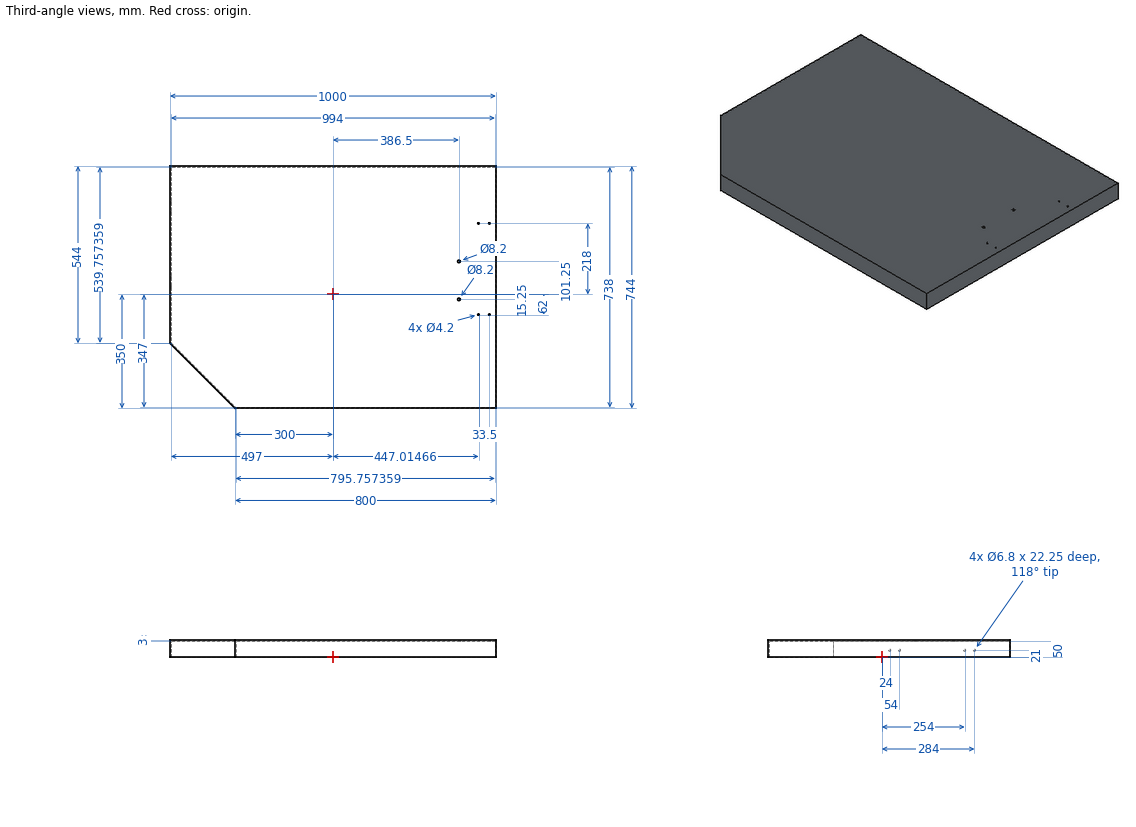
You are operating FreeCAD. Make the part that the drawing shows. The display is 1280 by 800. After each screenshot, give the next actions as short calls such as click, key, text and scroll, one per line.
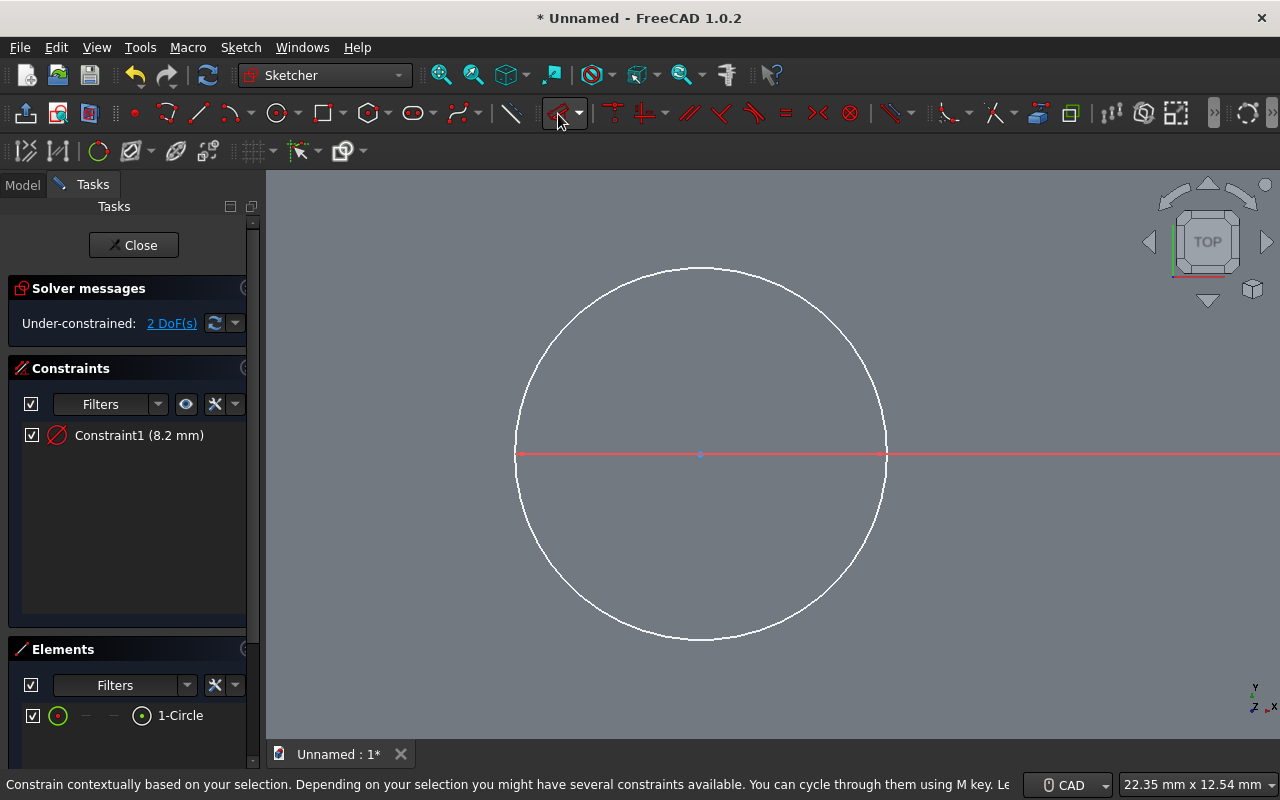
click(701, 454)
click(497, 420)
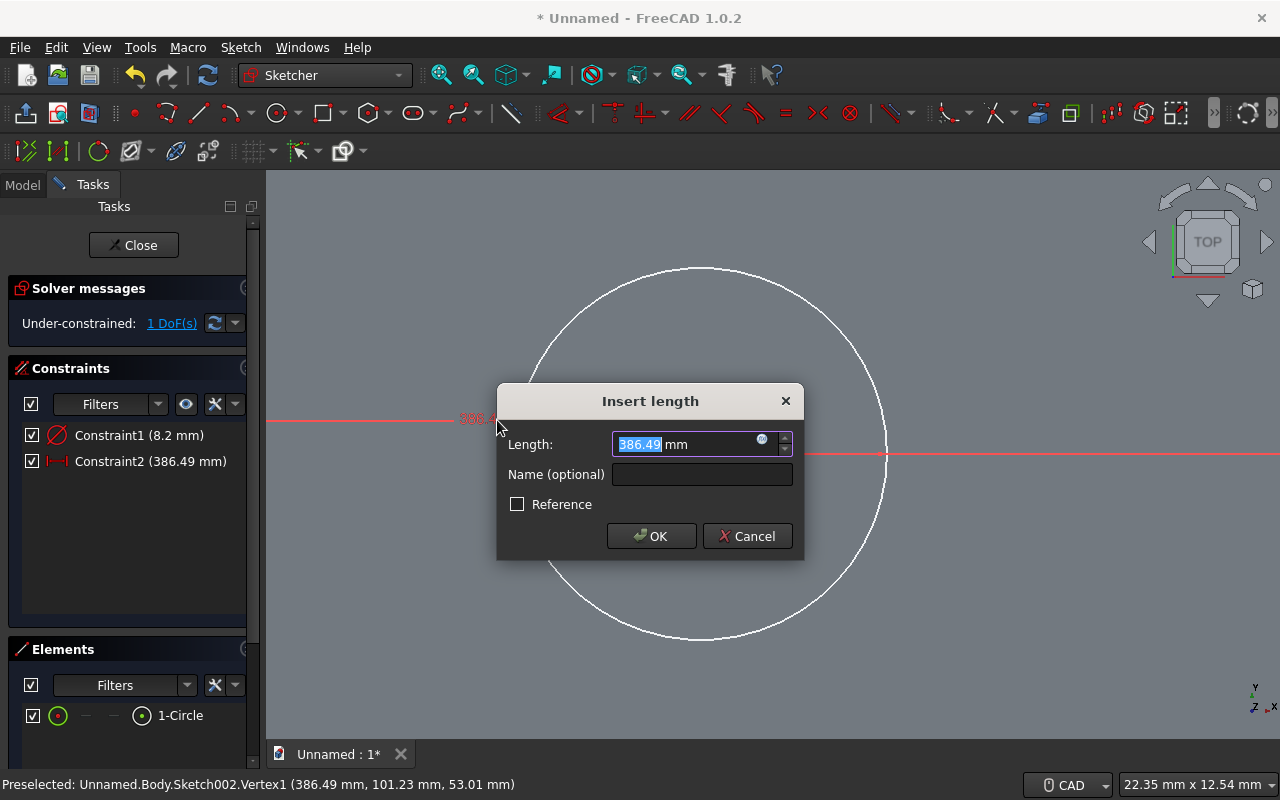
text(386.5)
key(Return)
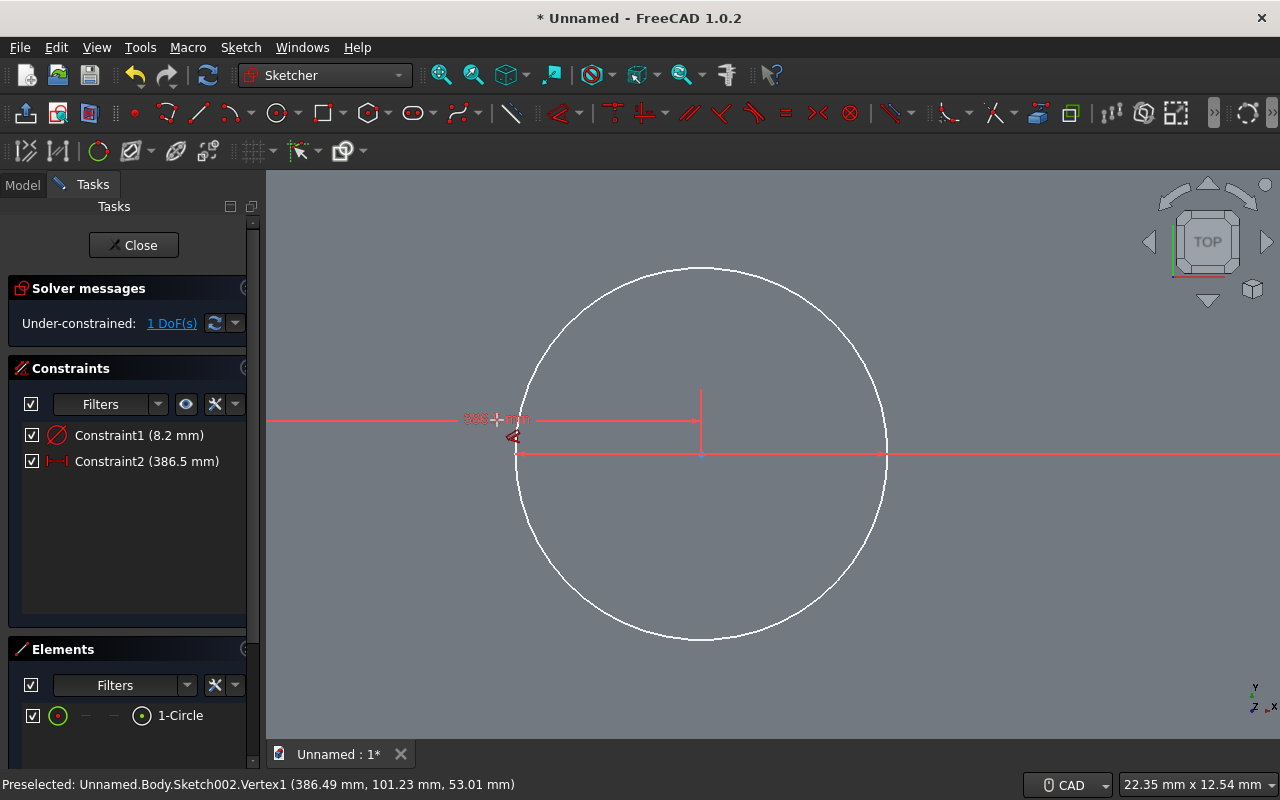
click(701, 454)
click(735, 583)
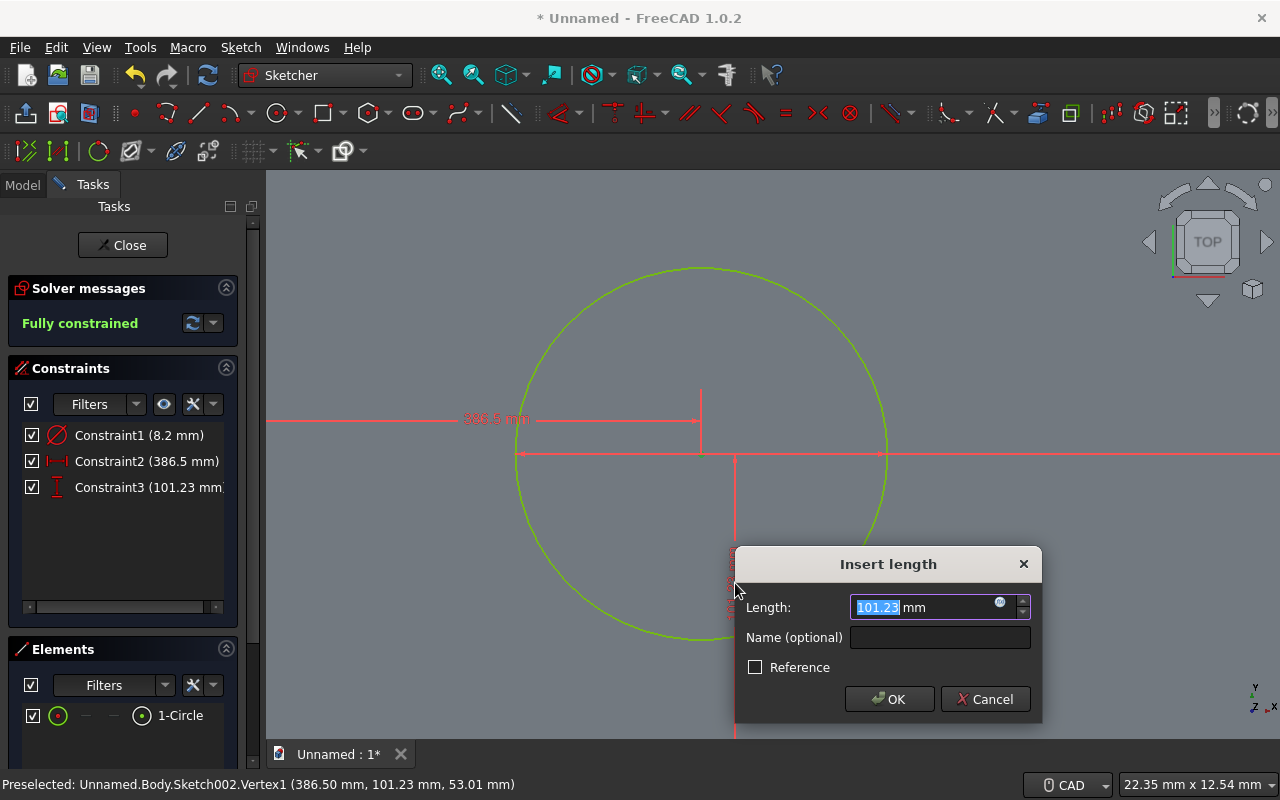
text(101.25)
key(Return)
key(Escape)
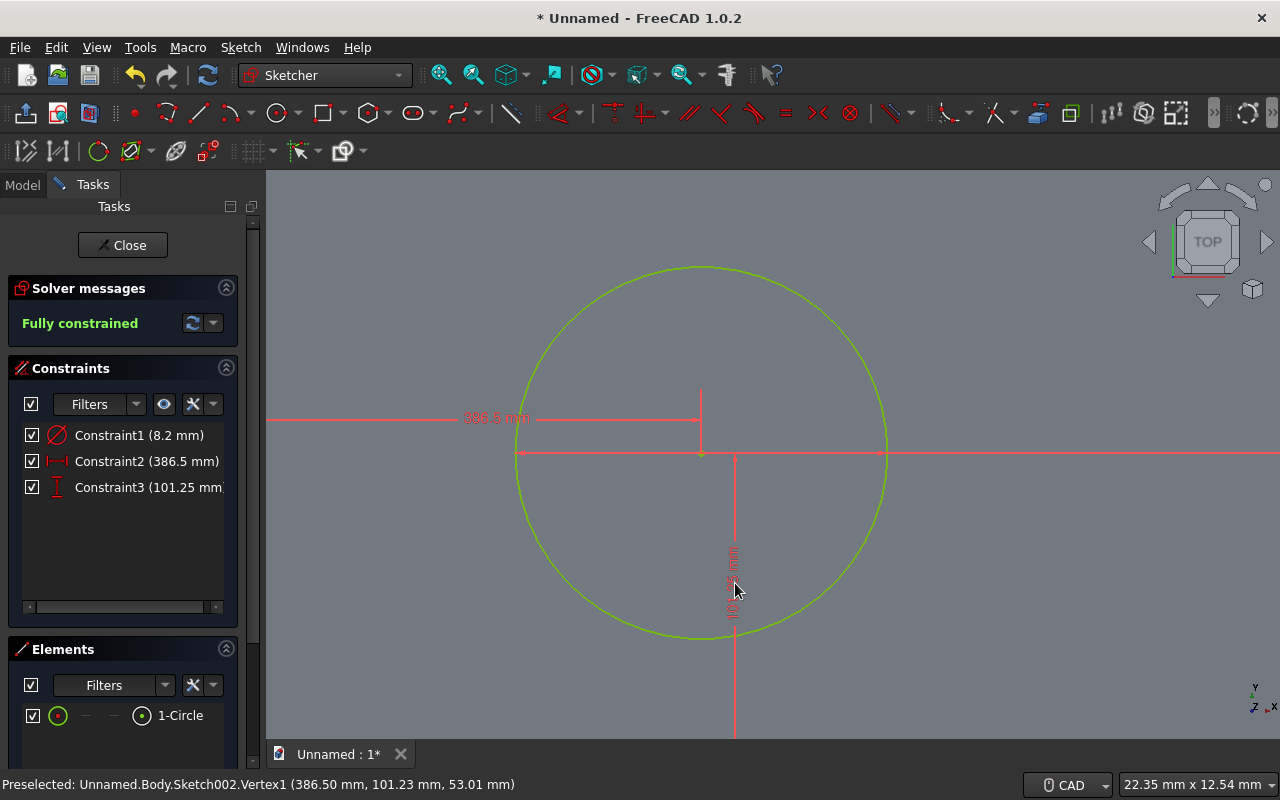
click(123, 245)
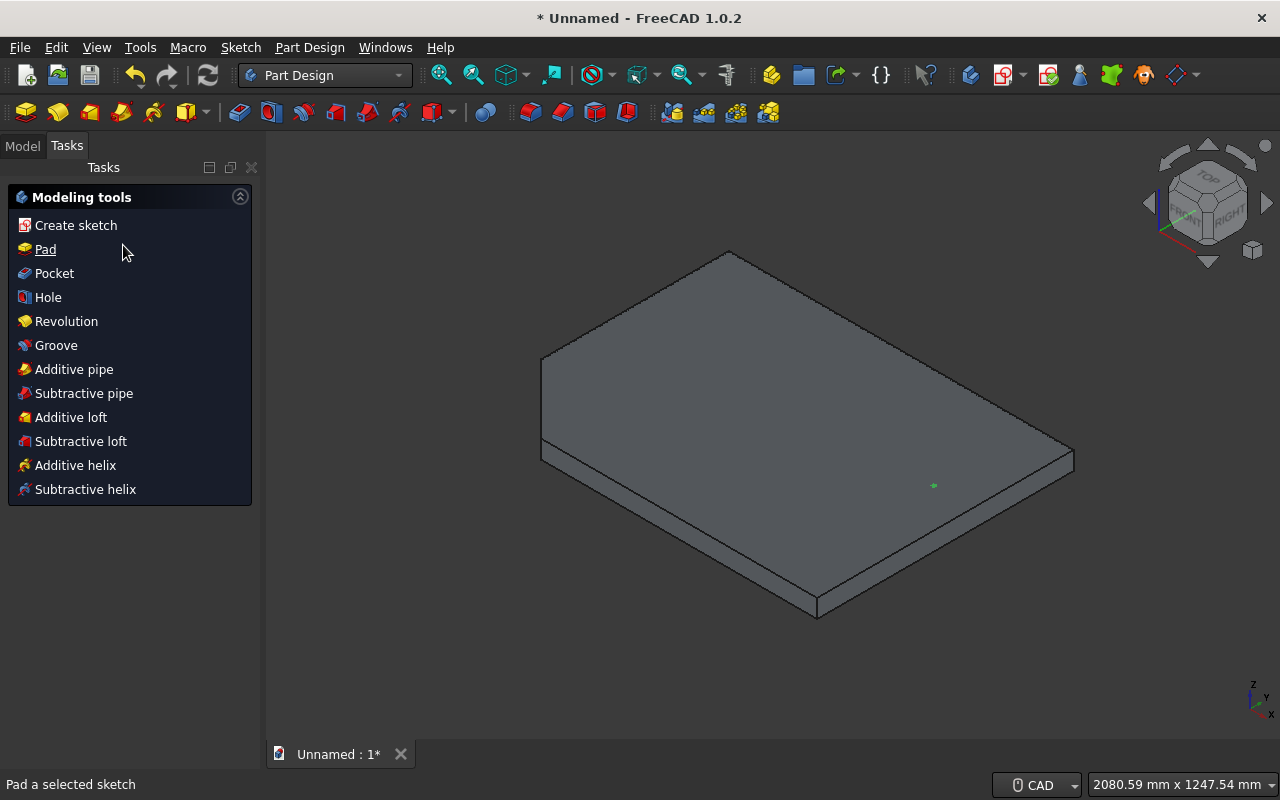
click(240, 112)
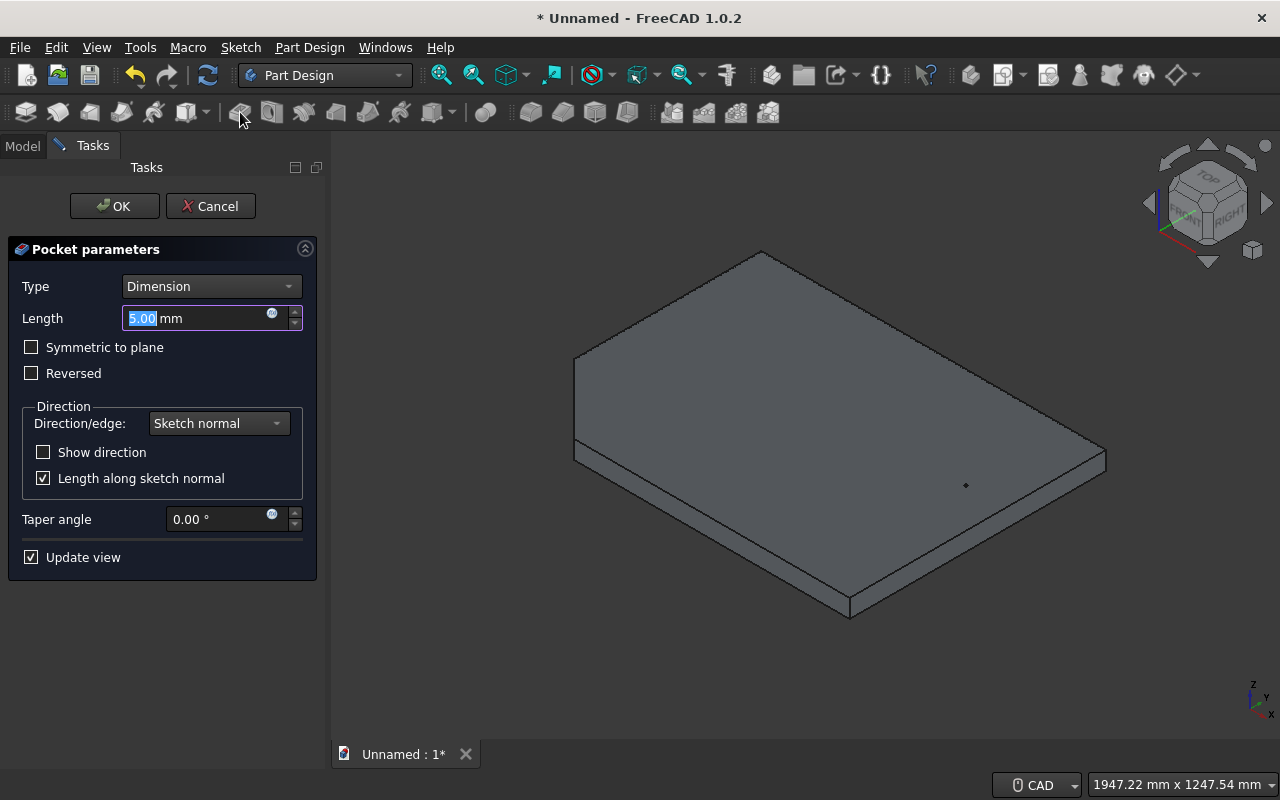
click(212, 286)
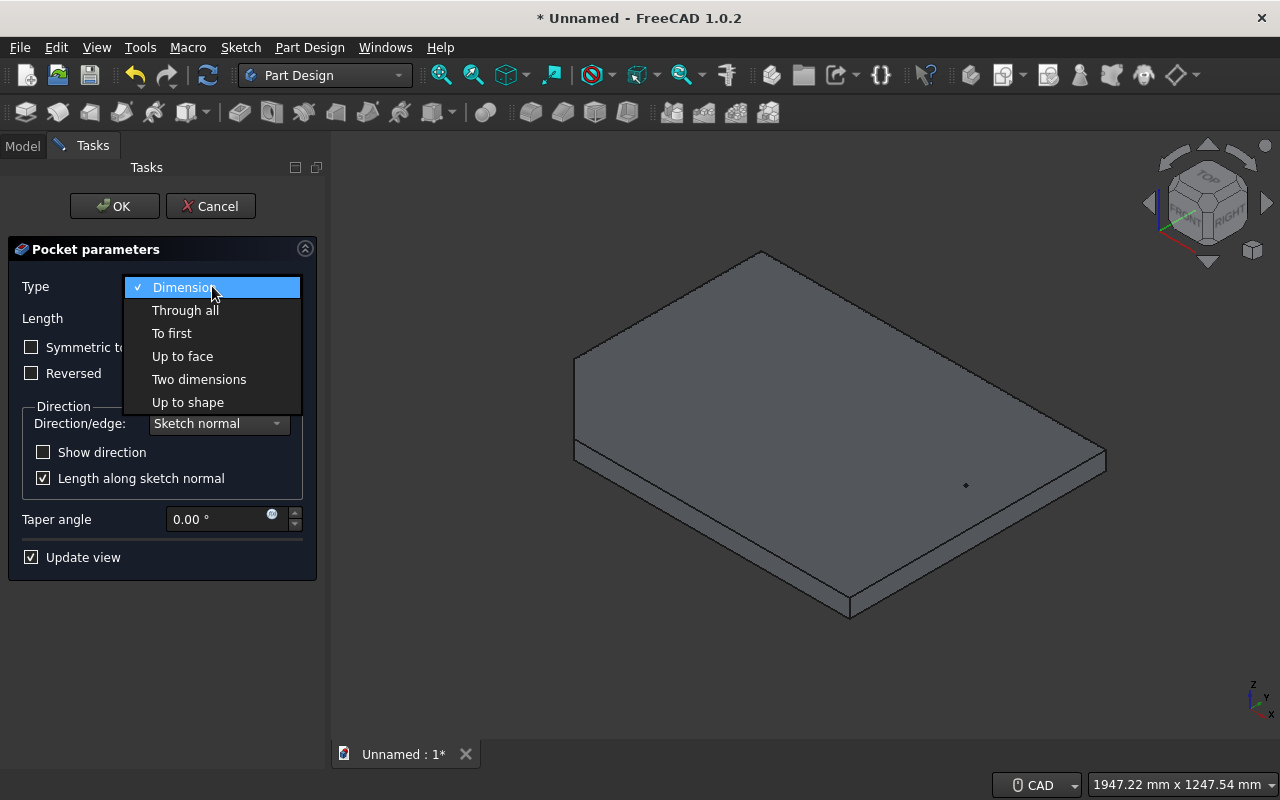
click(212, 334)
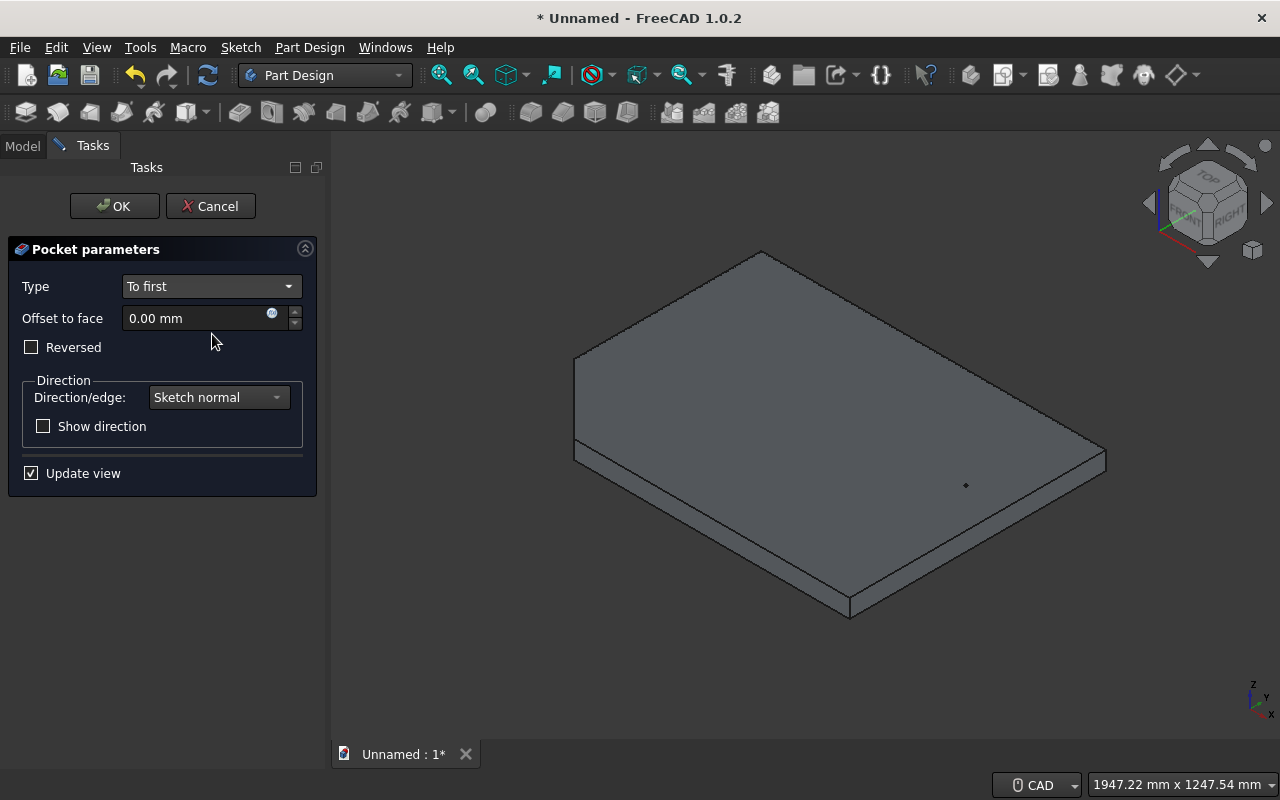
click(115, 206)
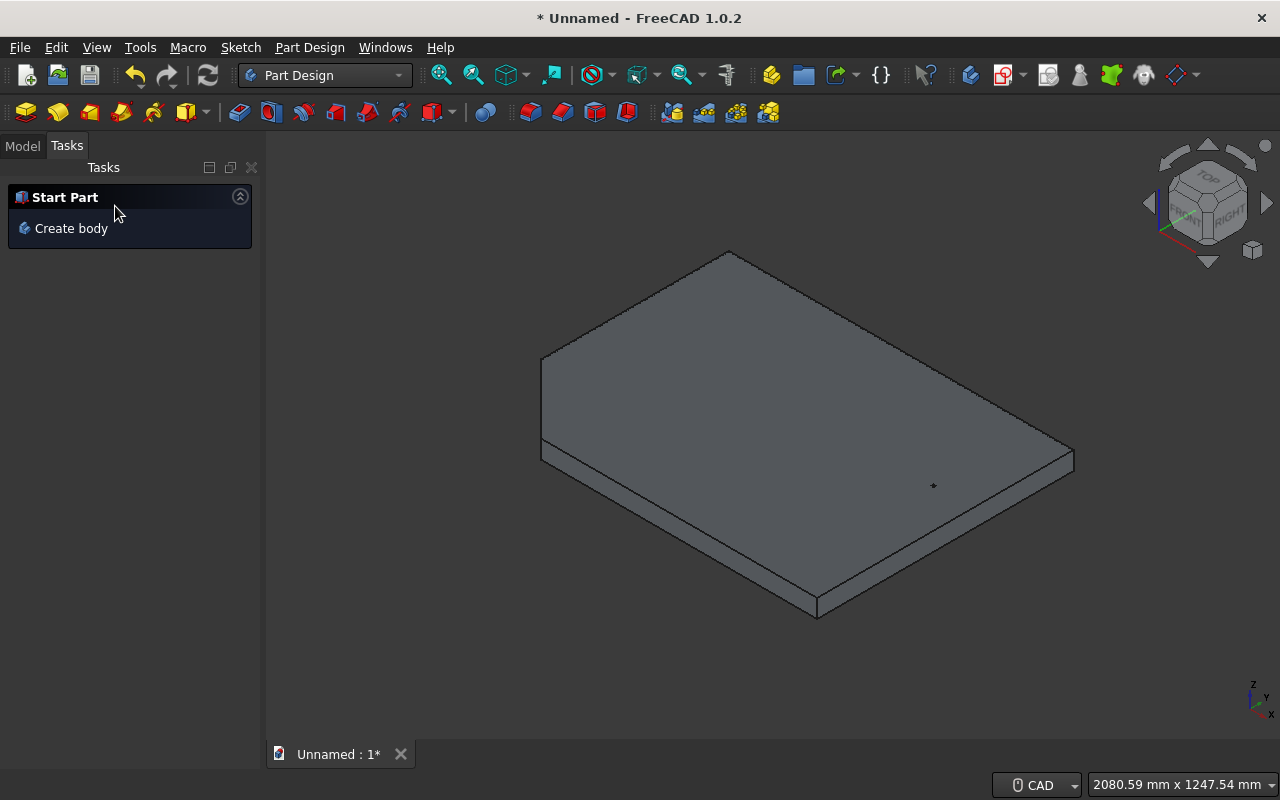
click(773, 423)